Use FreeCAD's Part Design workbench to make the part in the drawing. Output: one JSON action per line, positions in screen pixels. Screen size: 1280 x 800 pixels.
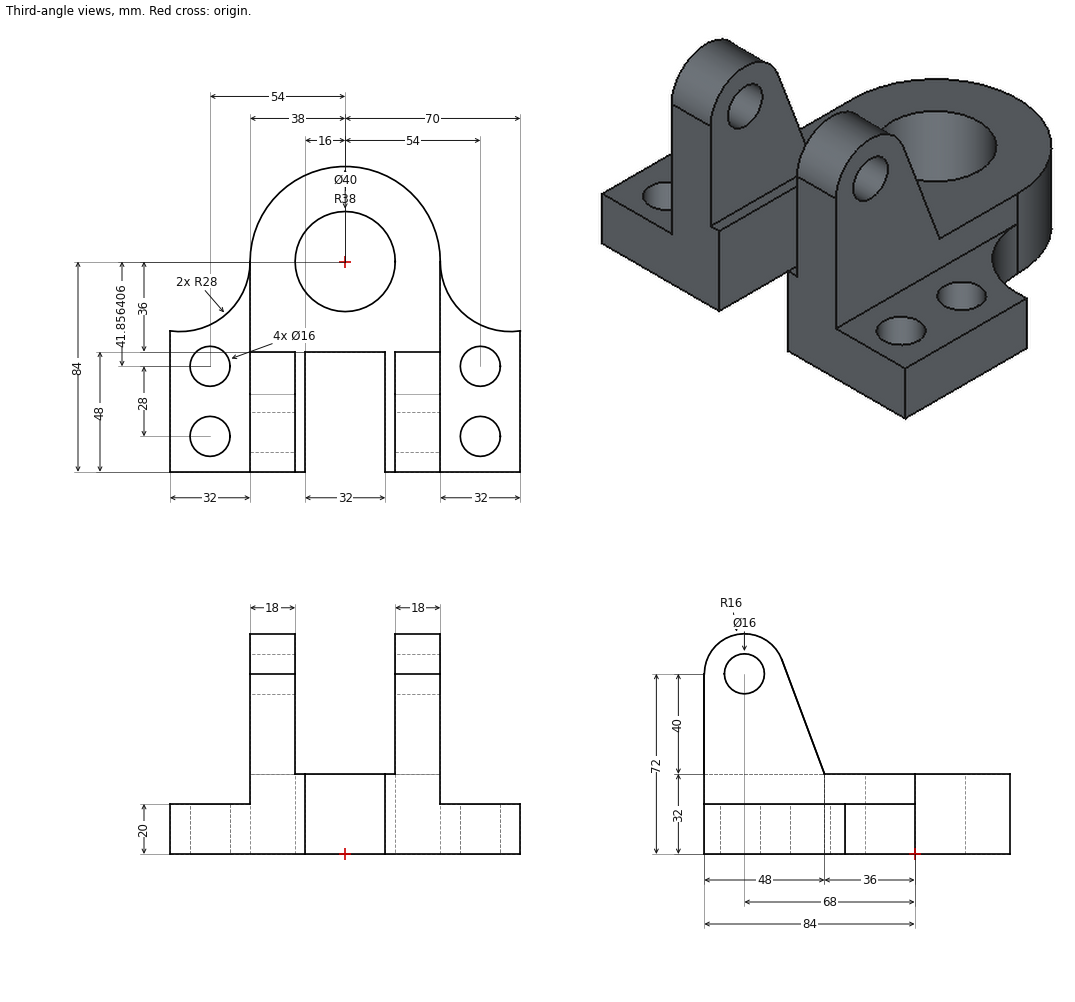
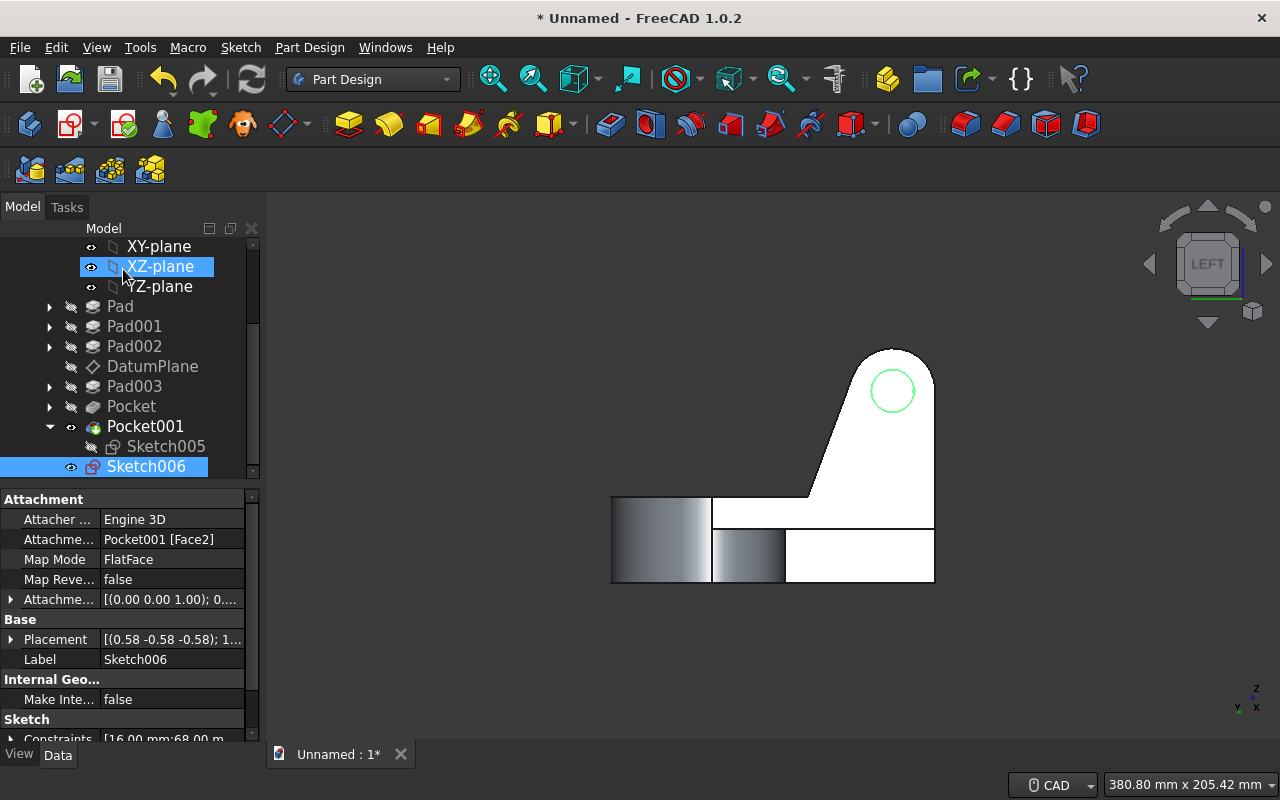
{"action": "left_click", "coordinate": [612, 124]}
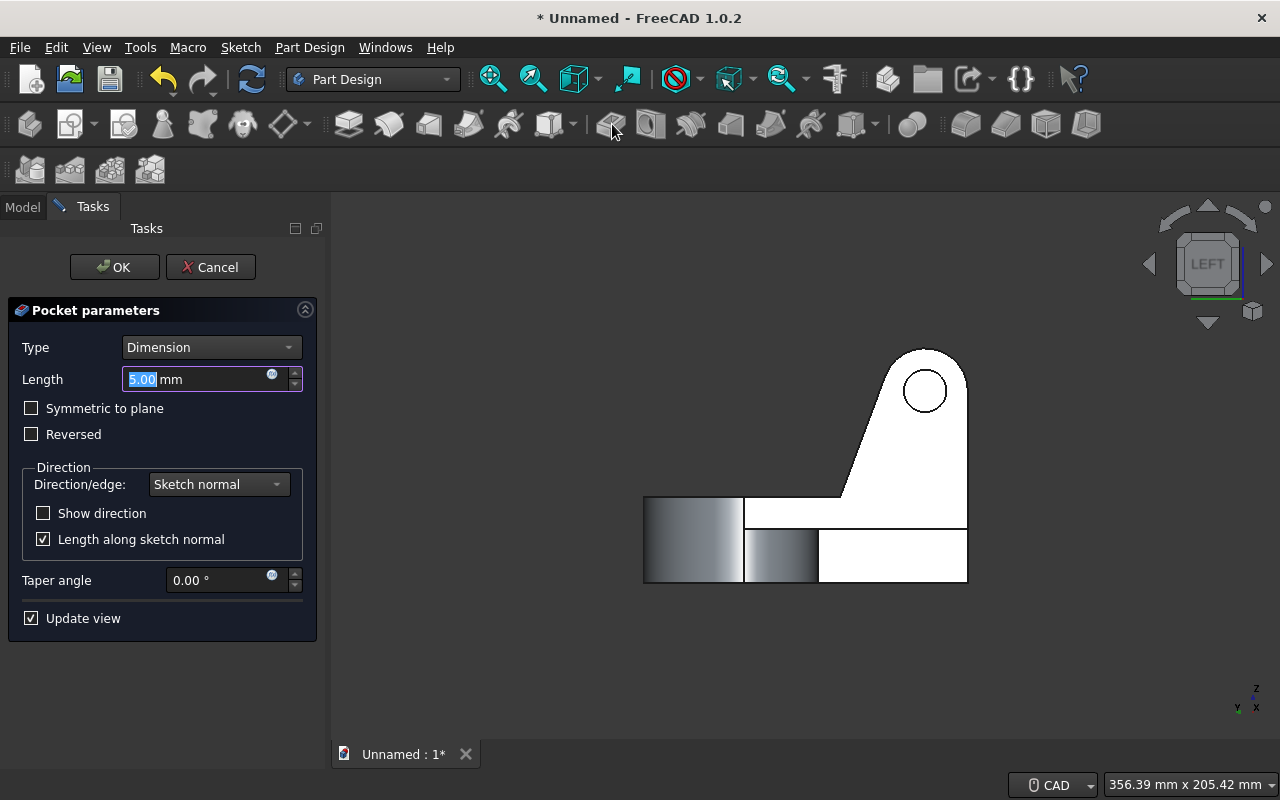
{"action": "left_click", "coordinate": [212, 348]}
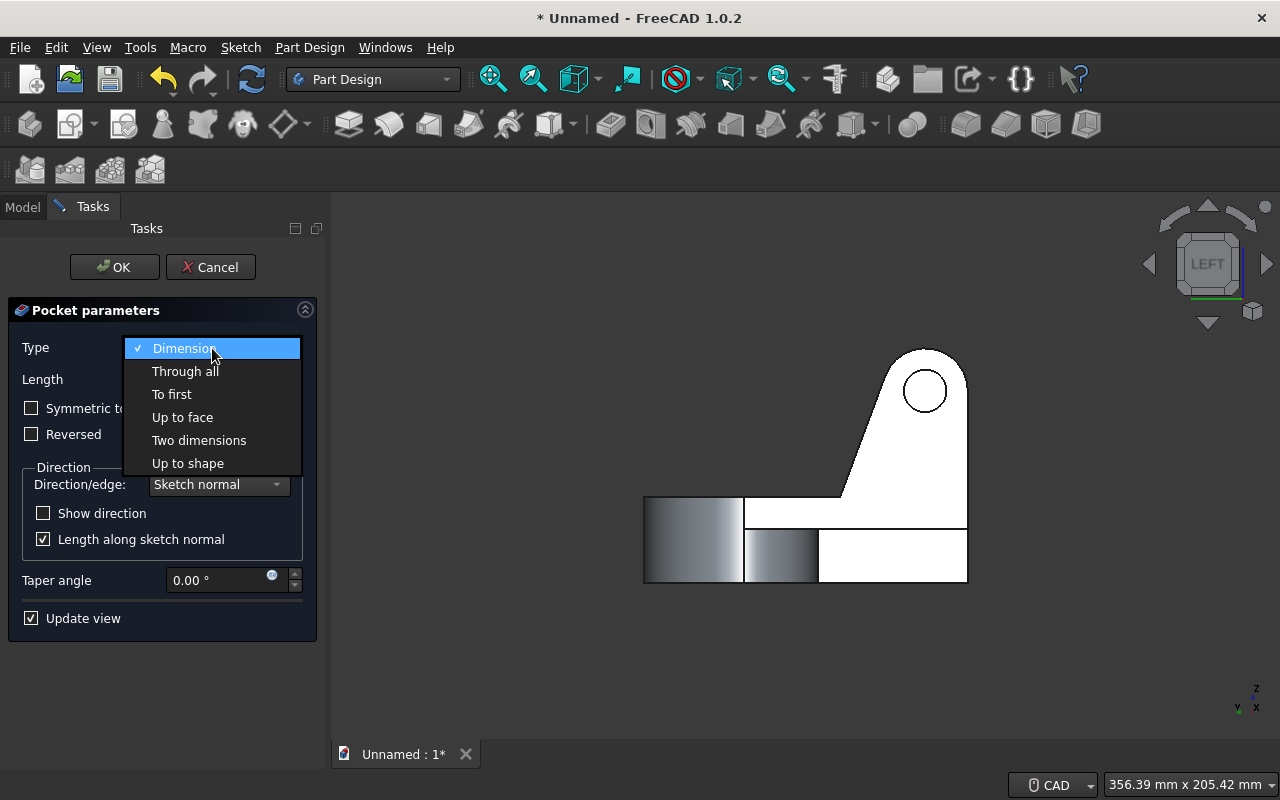
{"action": "left_click", "coordinate": [212, 372]}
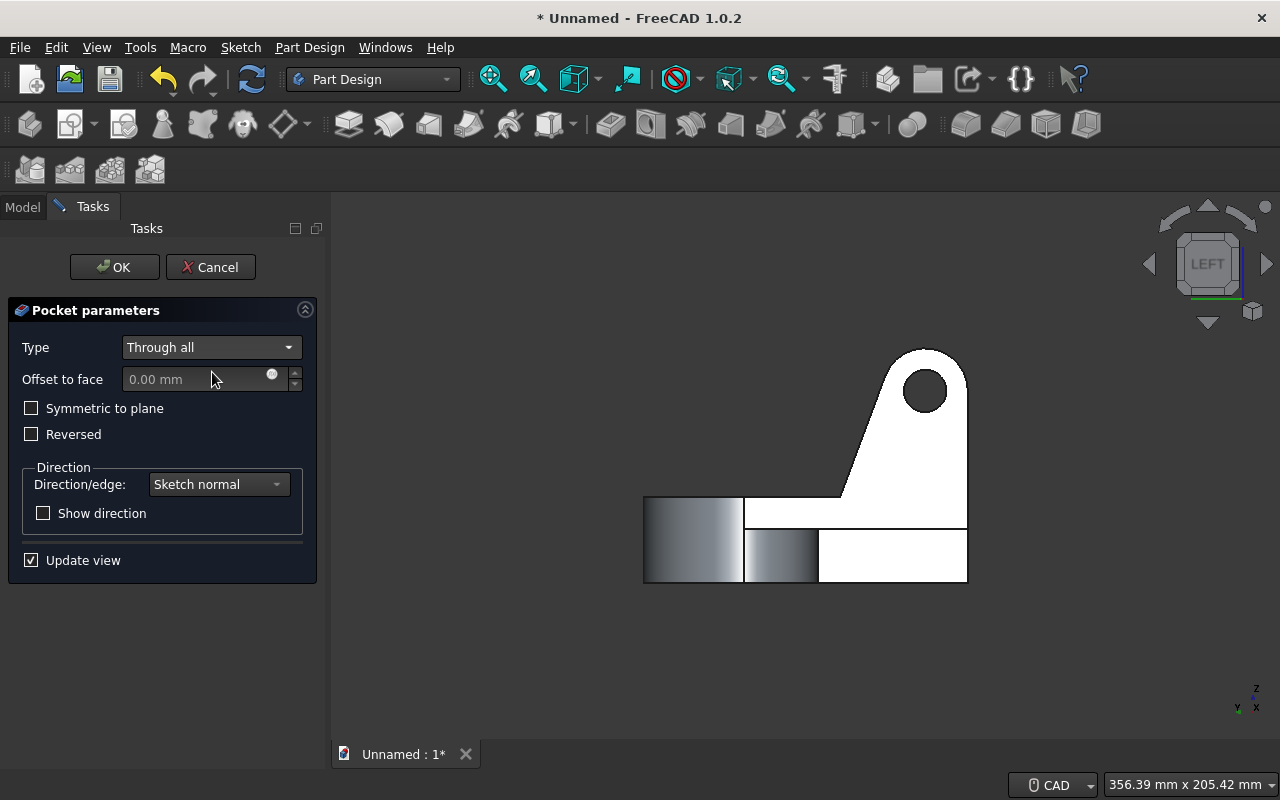
{"action": "left_click", "coordinate": [115, 267]}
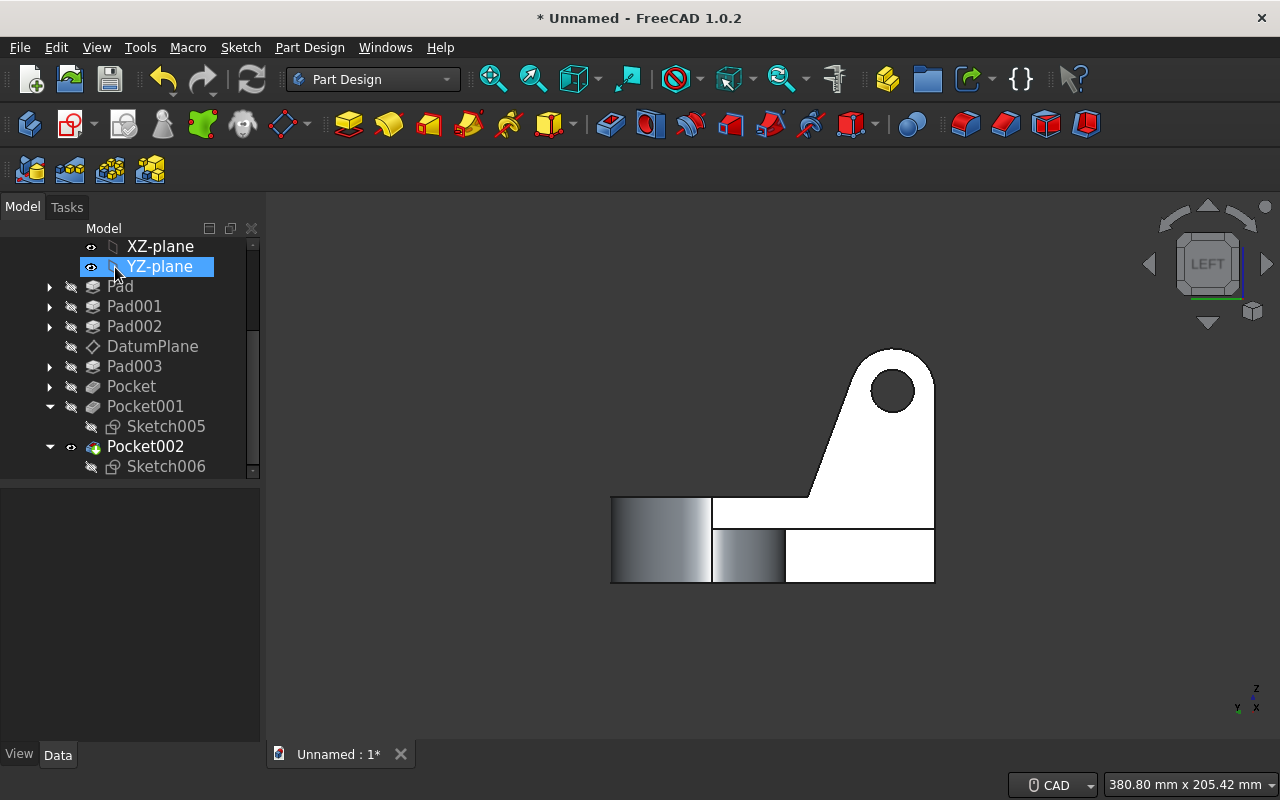
{"action": "left_click", "coordinate": [494, 80]}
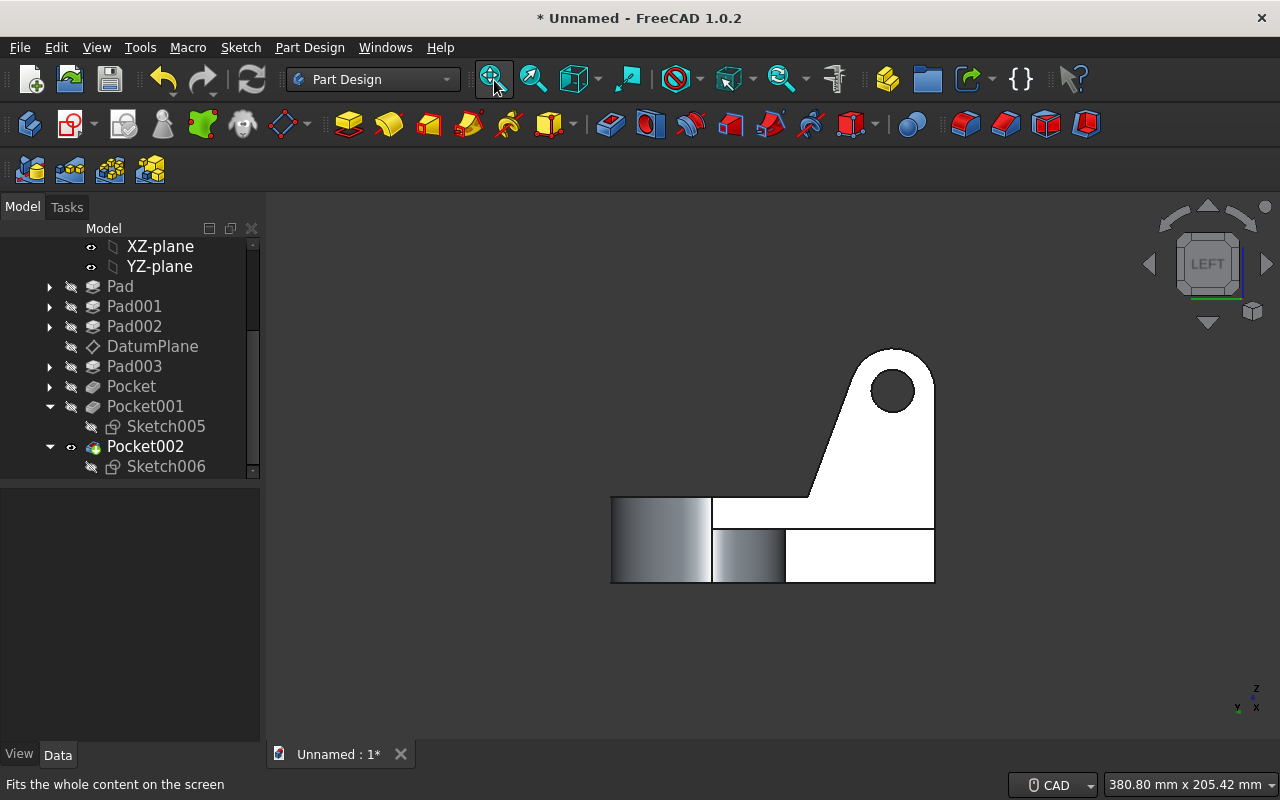
{"action": "key", "text": "0"}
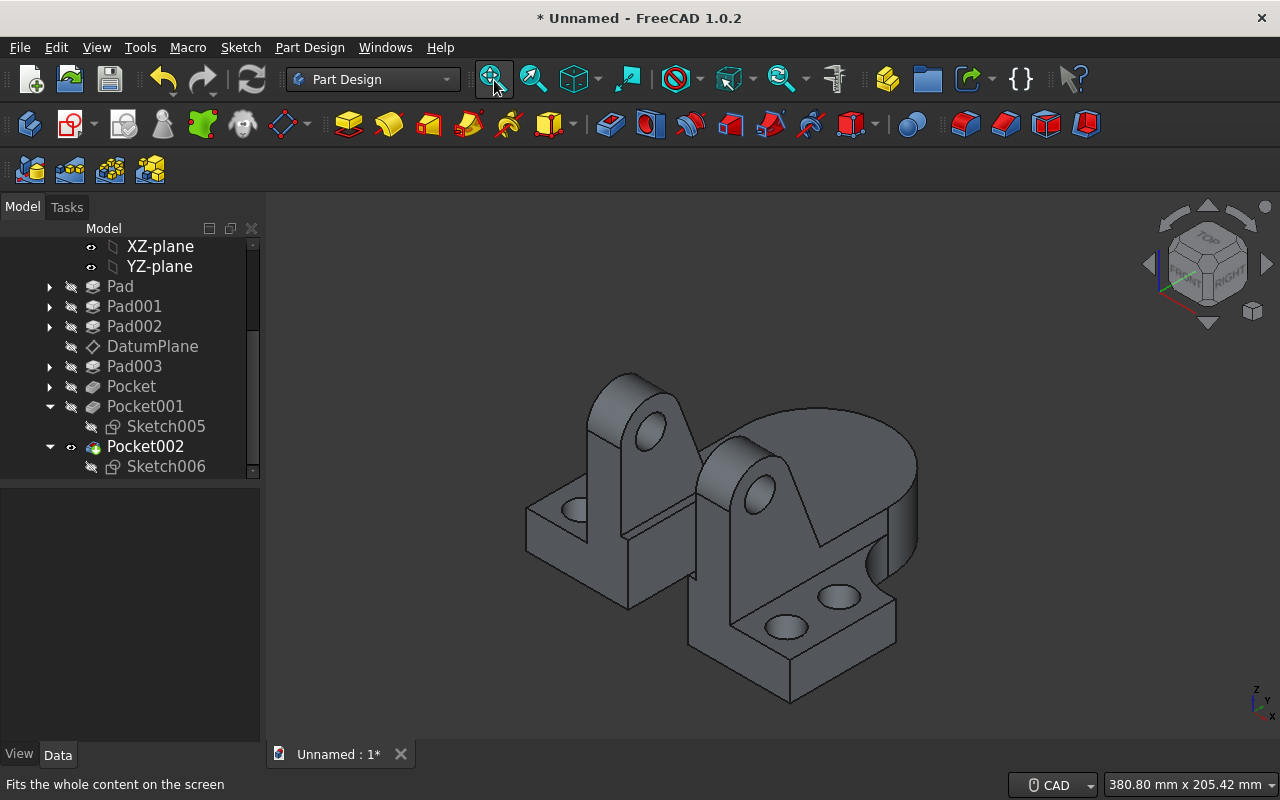
{"action": "left_click", "coordinate": [806, 472]}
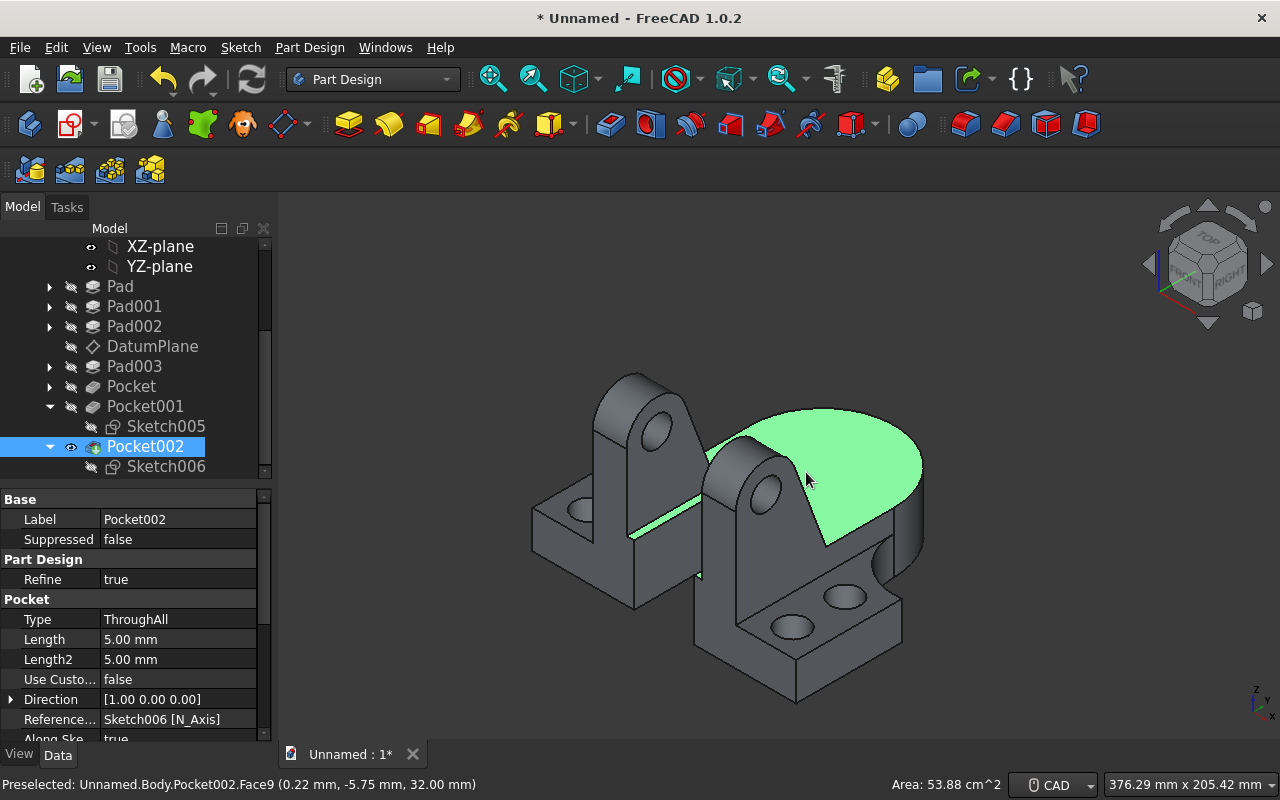
{"action": "left_click", "coordinate": [70, 124]}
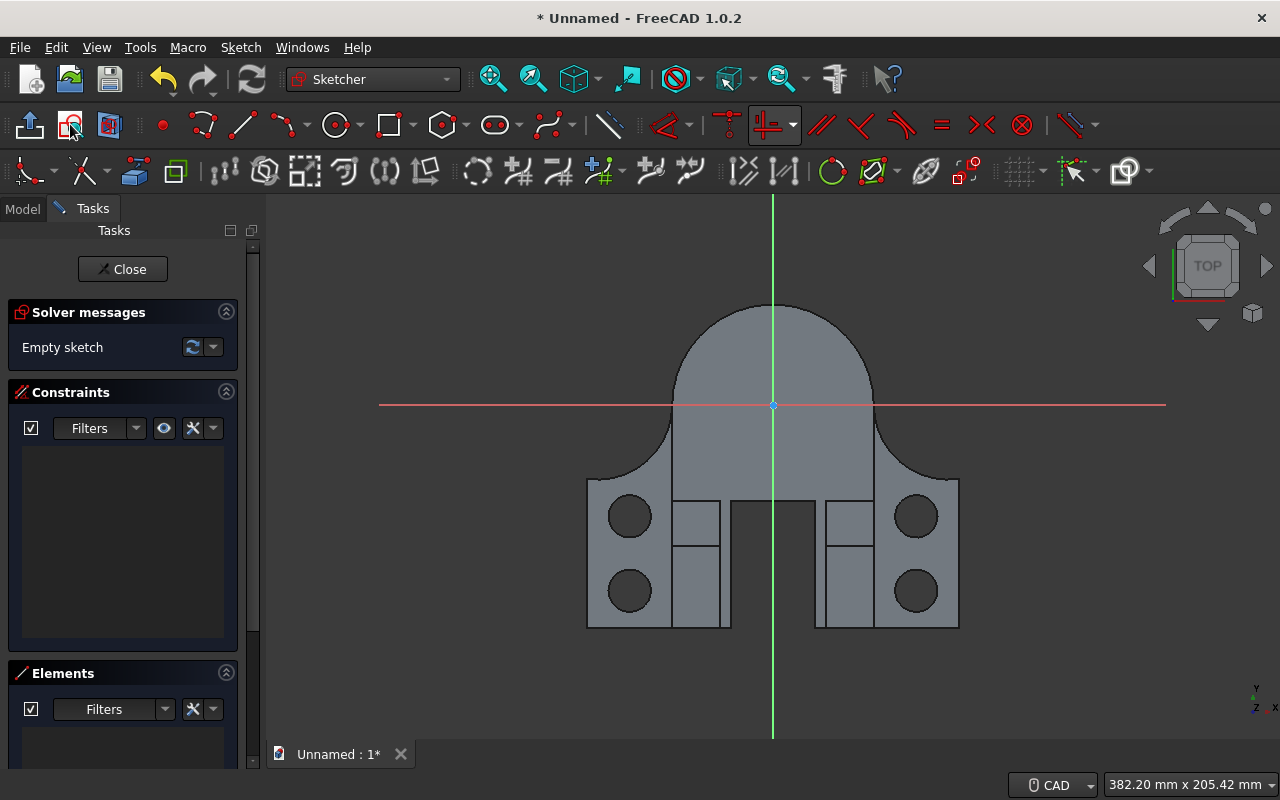
{"action": "left_click", "coordinate": [110, 126]}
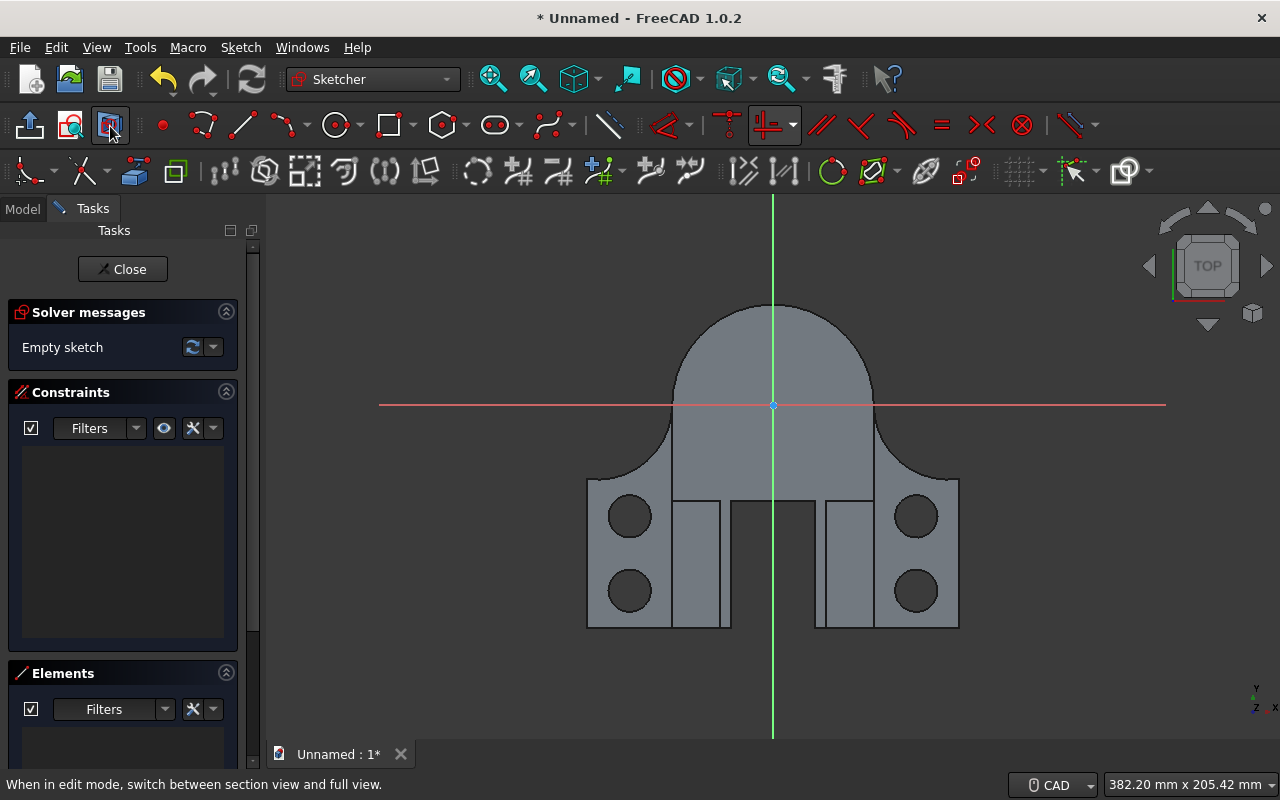
{"action": "scroll", "coordinate": [803, 379], "scroll_direction": "up", "scroll_amount": 6}